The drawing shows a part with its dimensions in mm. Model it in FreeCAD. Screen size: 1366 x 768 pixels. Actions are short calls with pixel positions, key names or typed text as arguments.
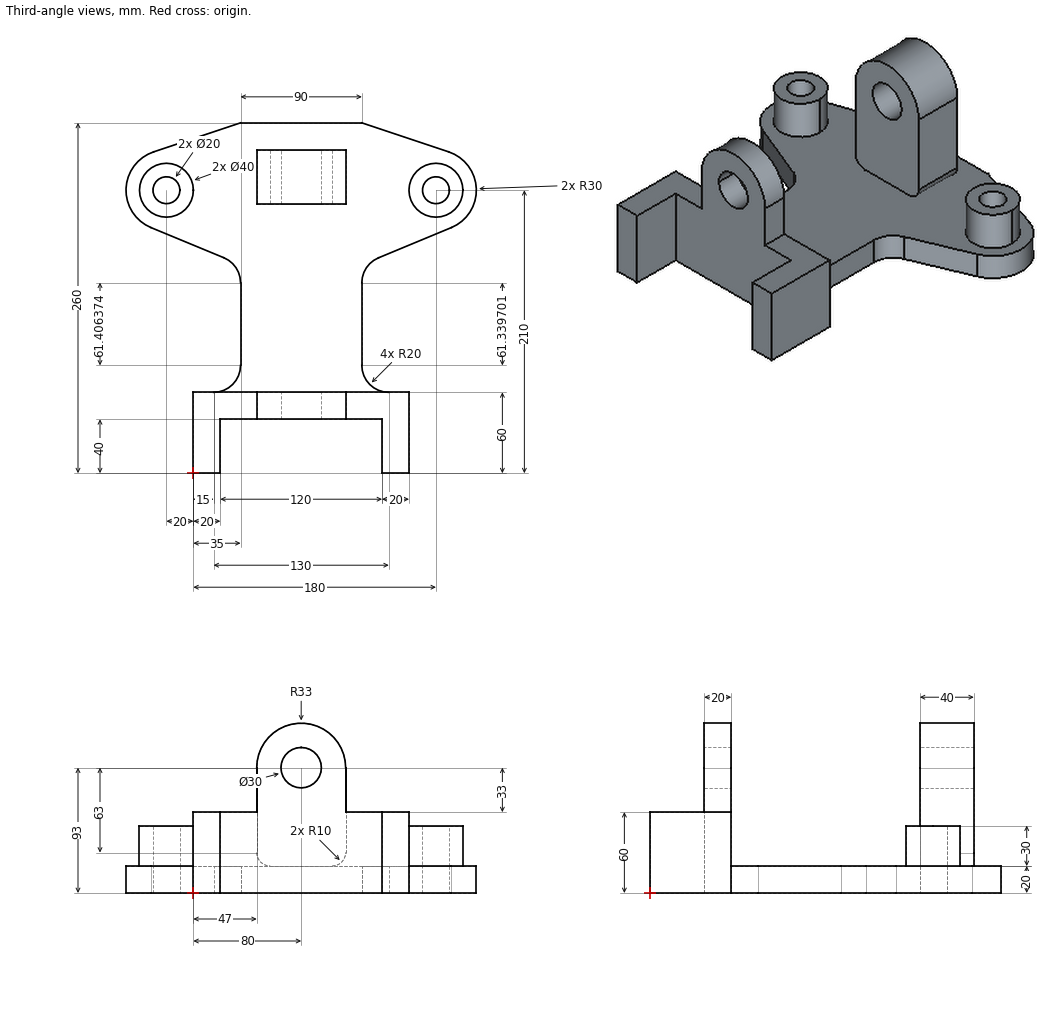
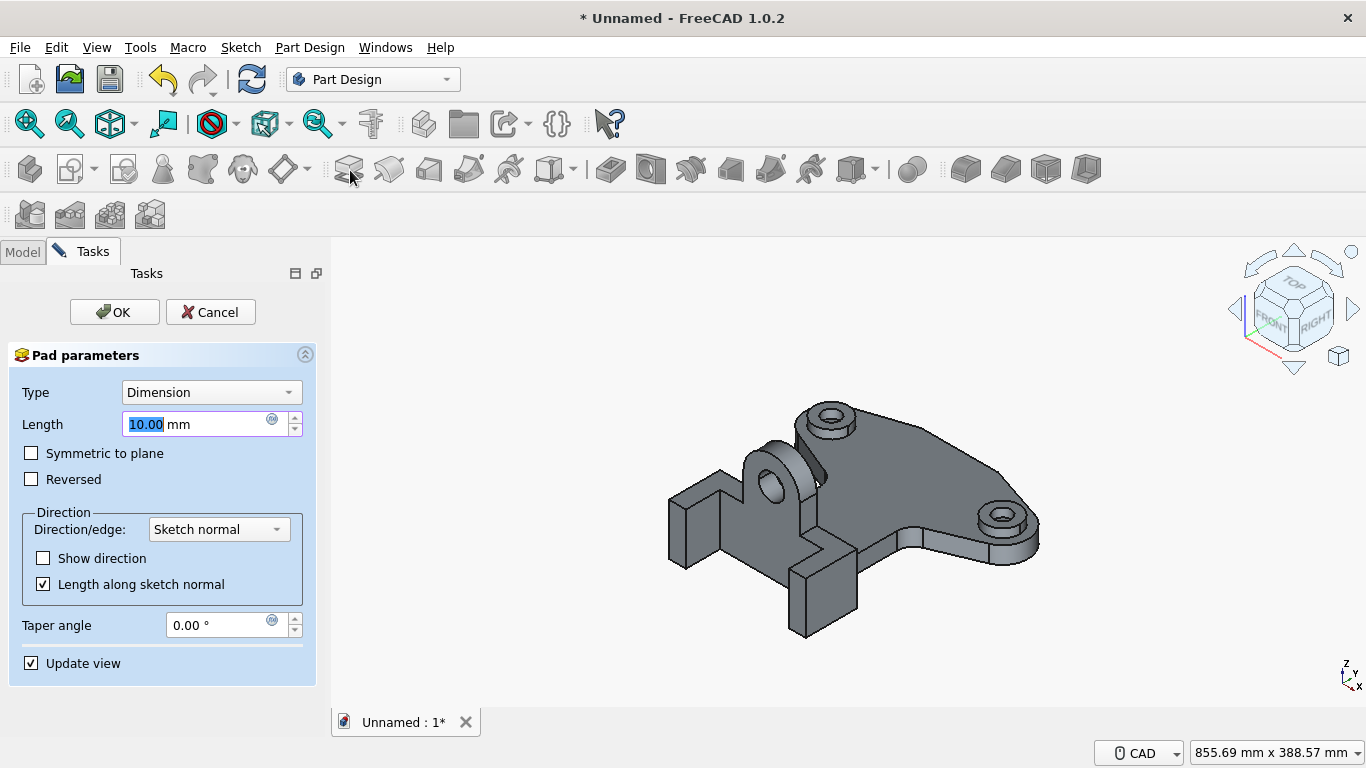
text(30)
key(Tab)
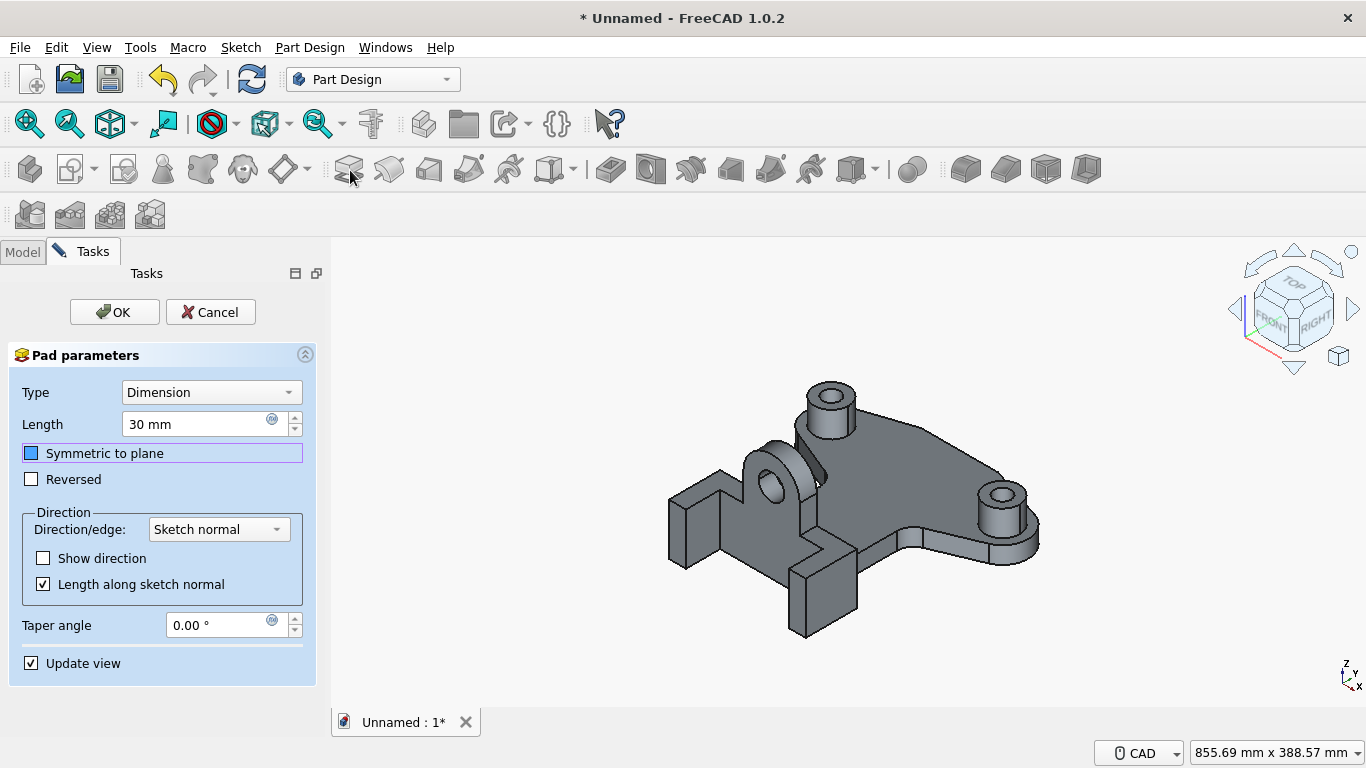
click(115, 312)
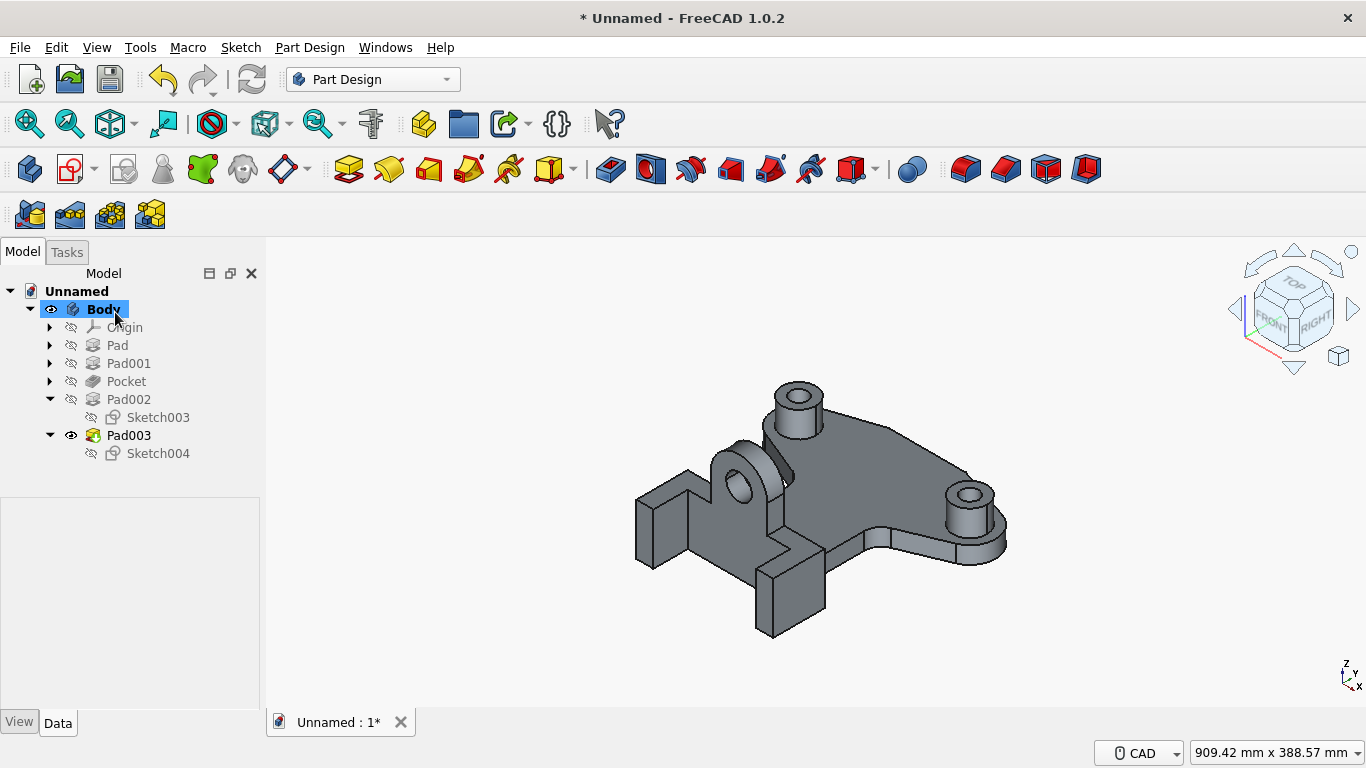
click(50, 327)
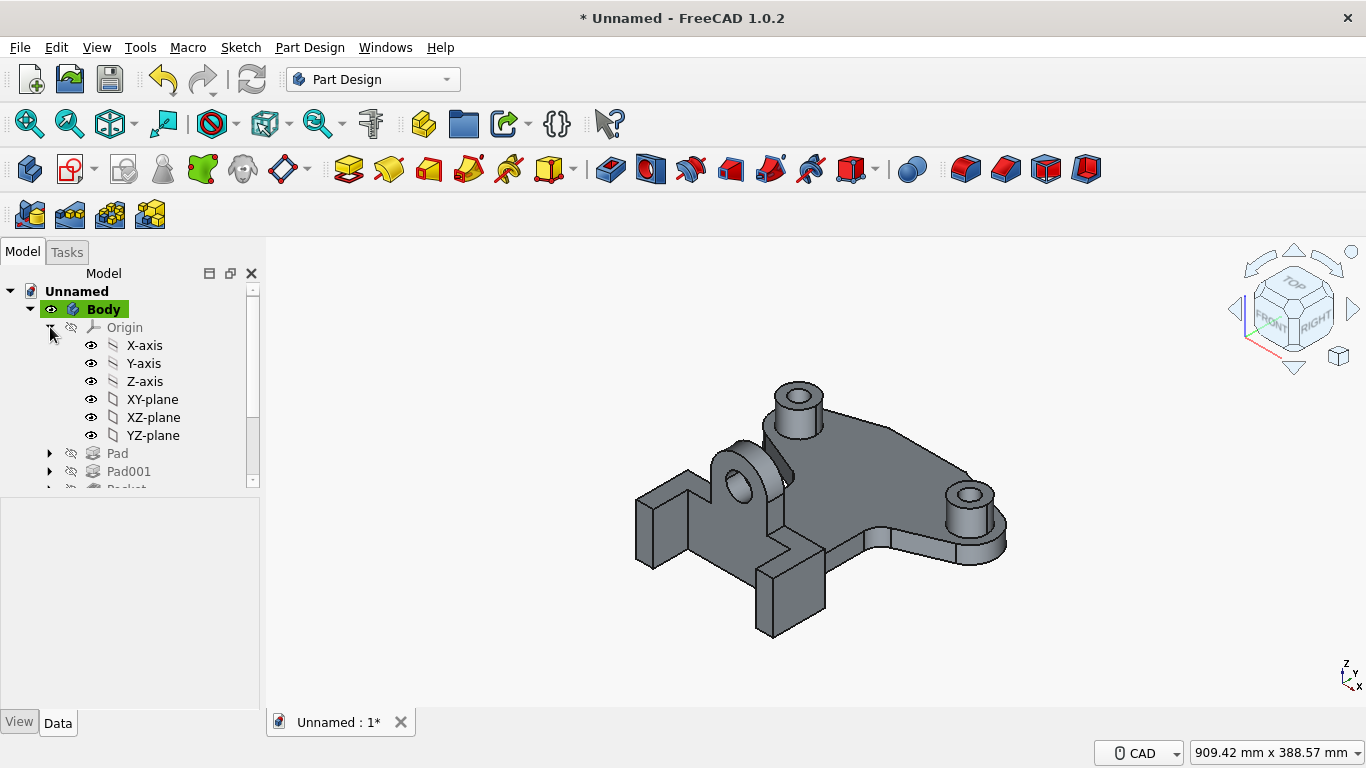
click(136, 417)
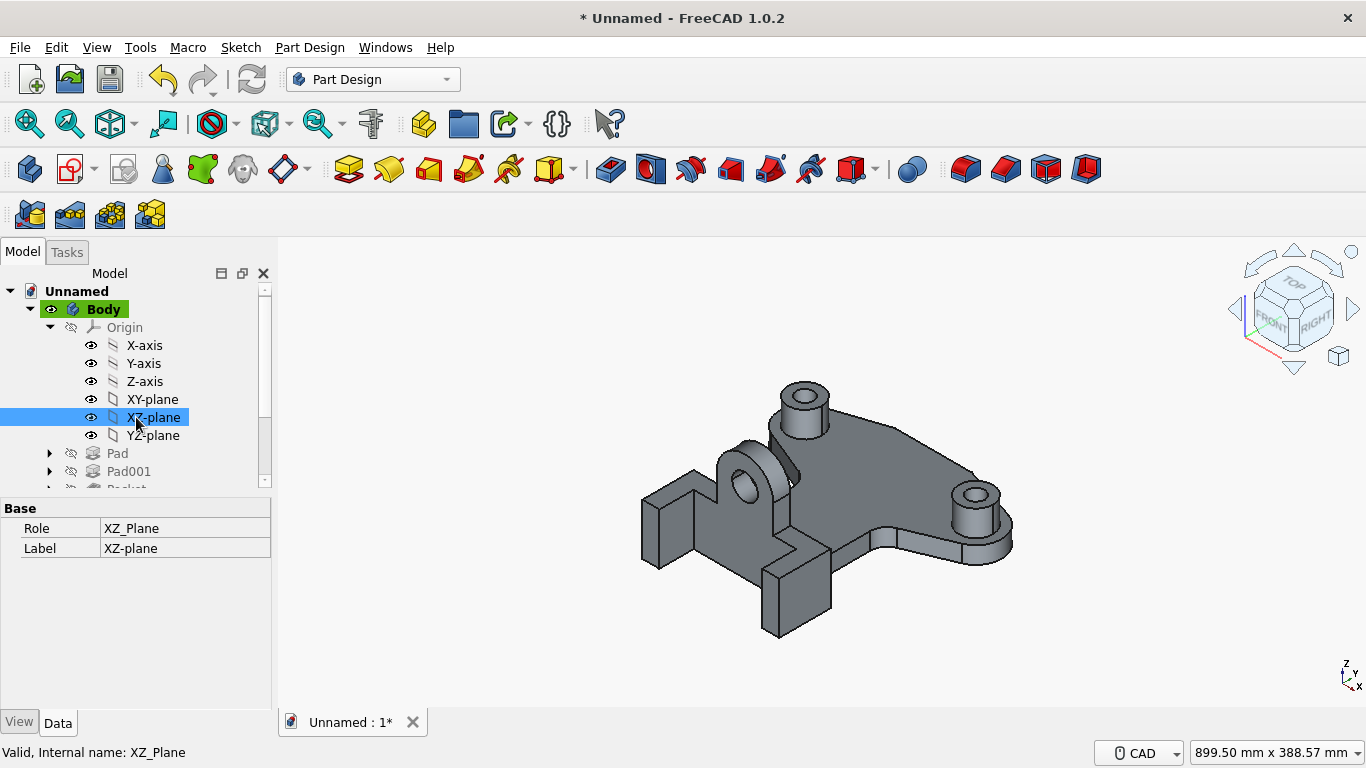
click(284, 170)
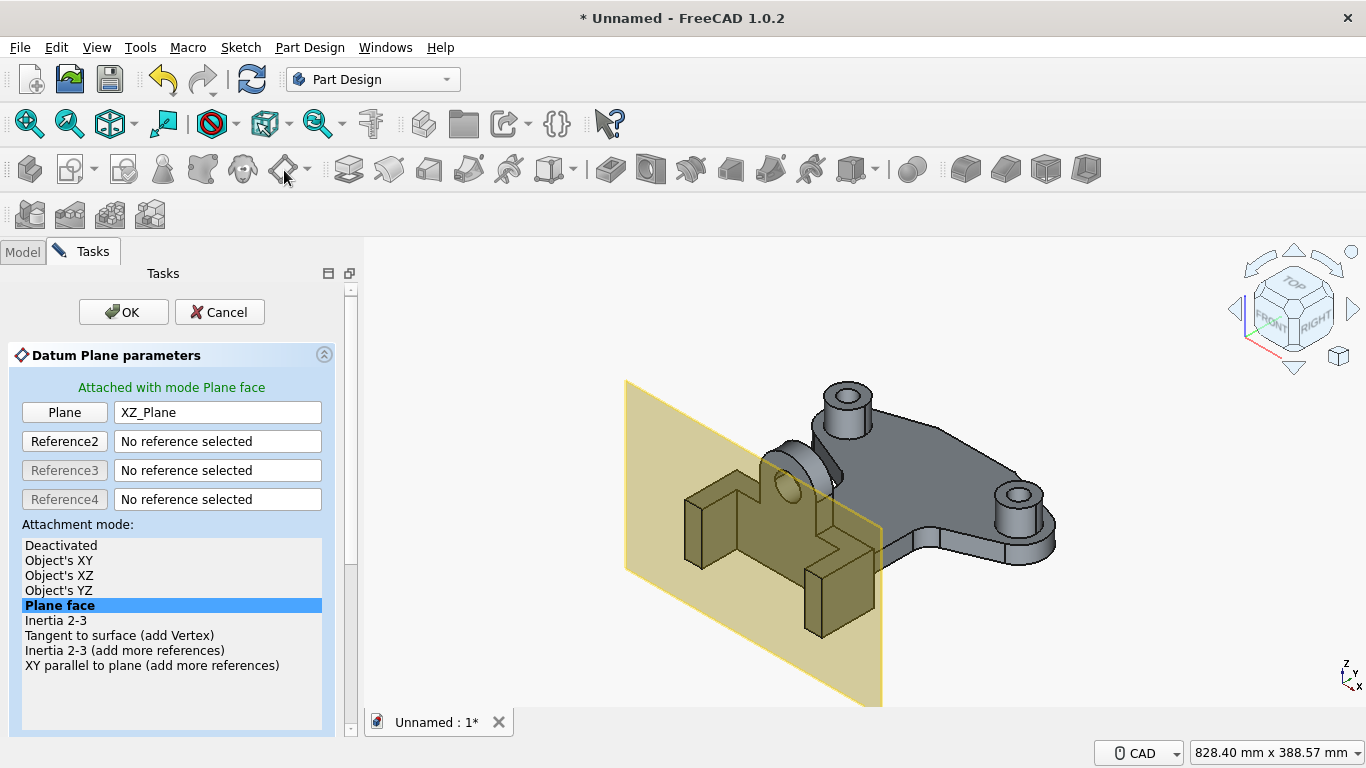
scroll(351, 510, down, 3)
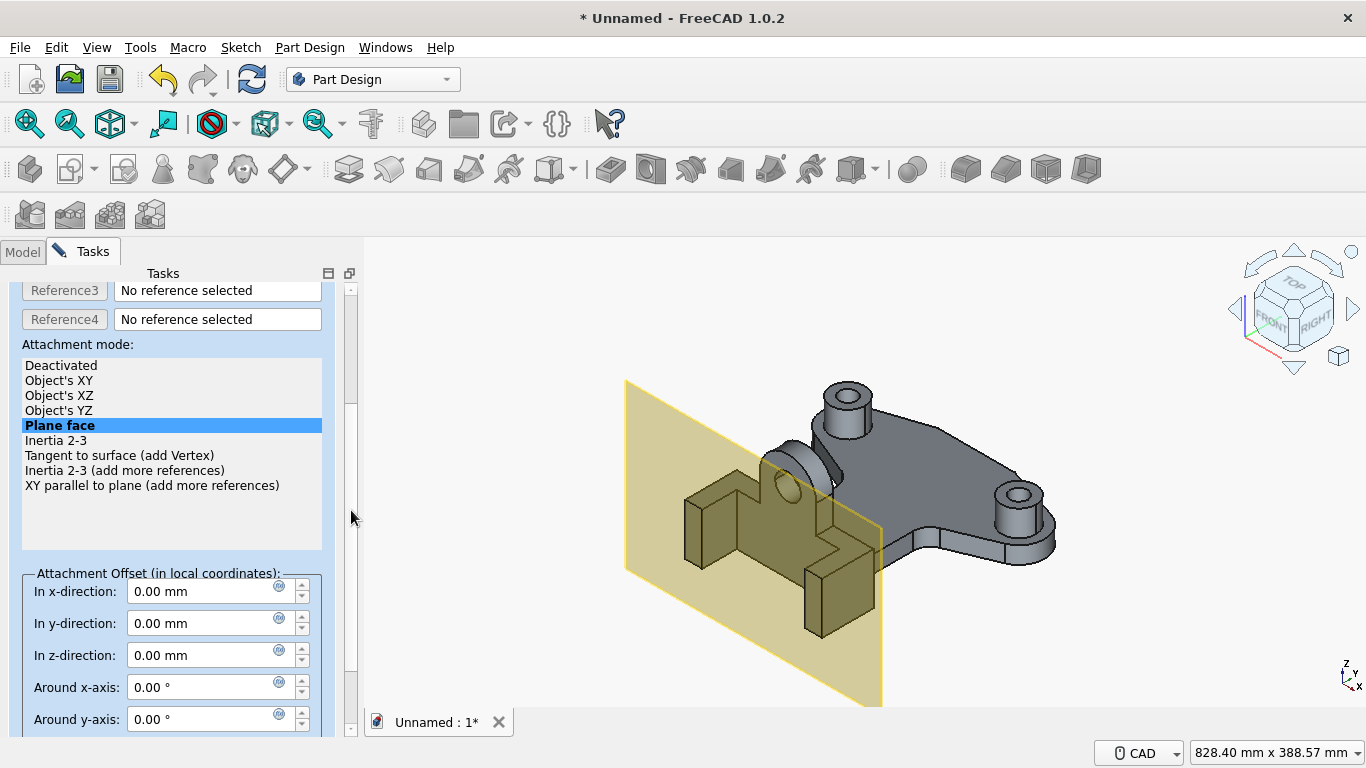
triple_click(210, 655)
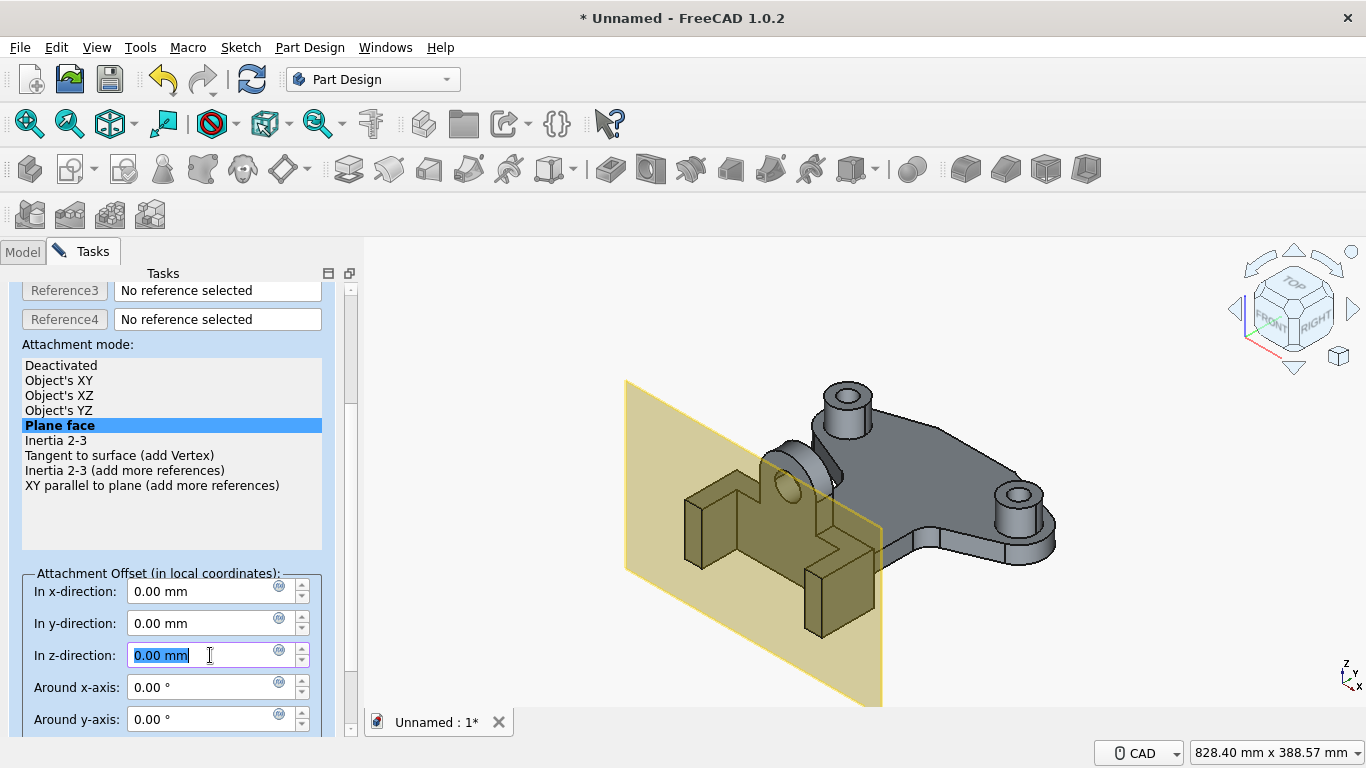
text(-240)
key(Tab)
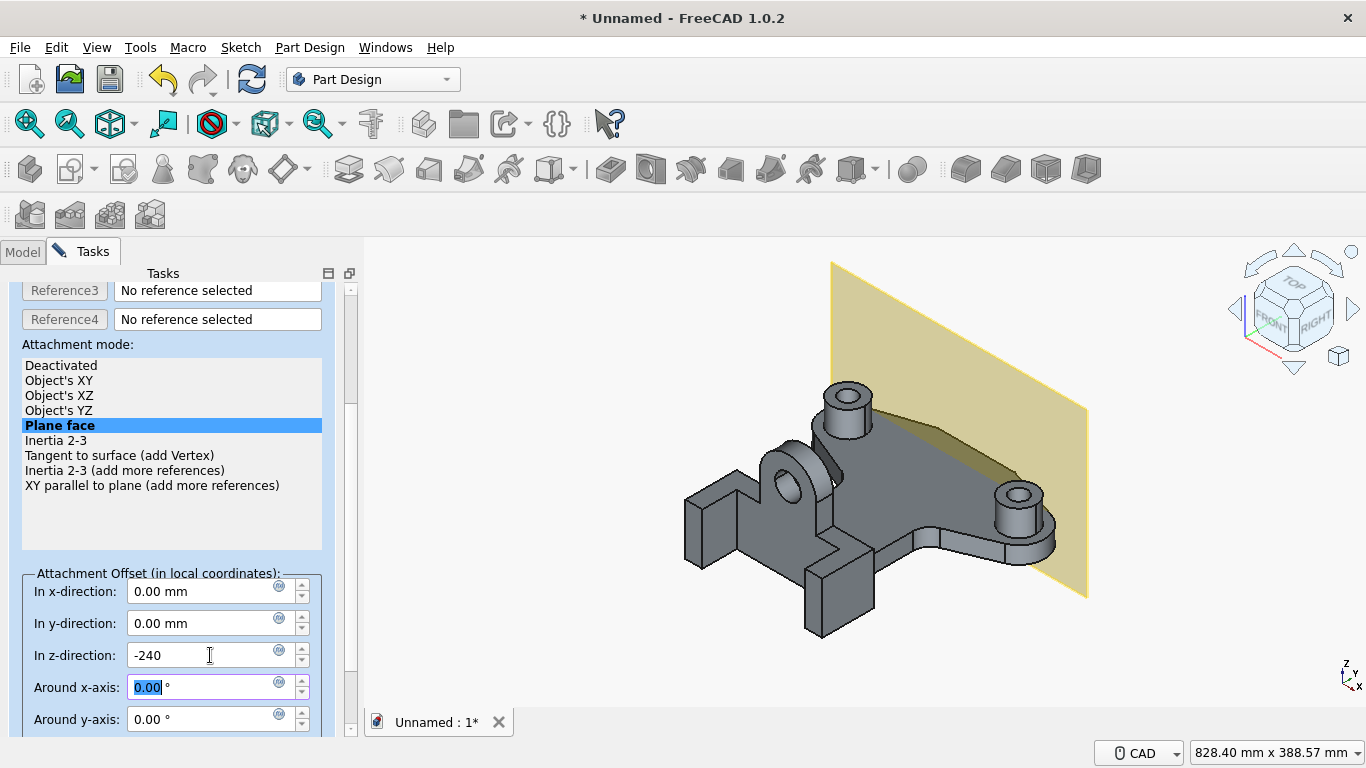
scroll(351, 510, up, 4)